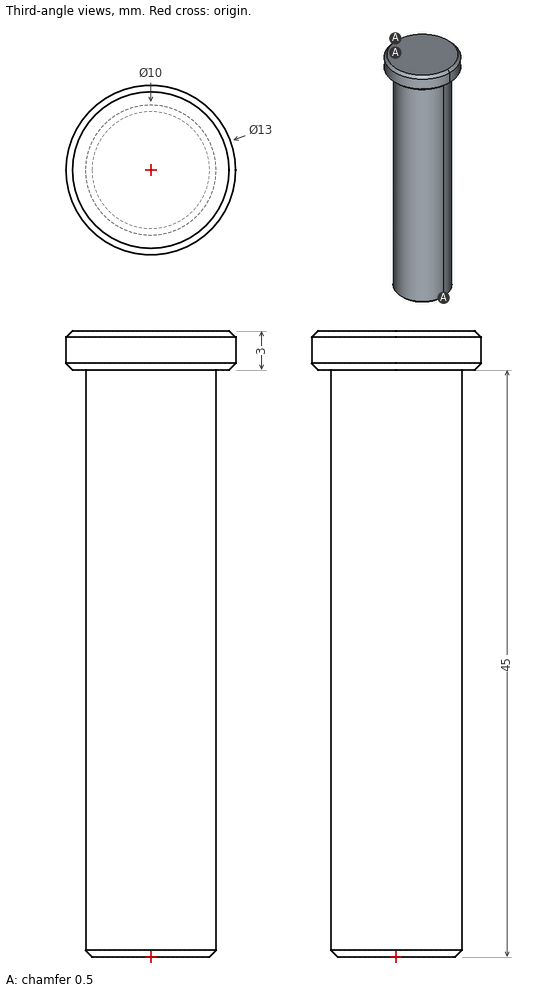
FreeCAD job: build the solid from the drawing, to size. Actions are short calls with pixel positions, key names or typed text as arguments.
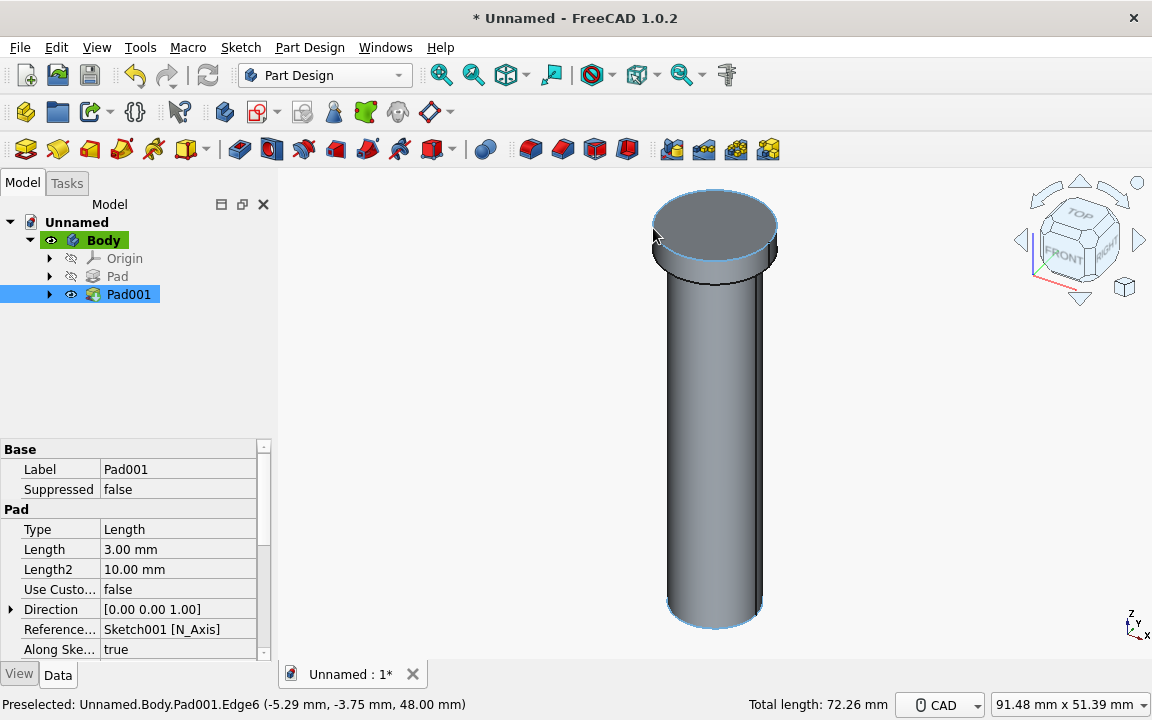
key(0)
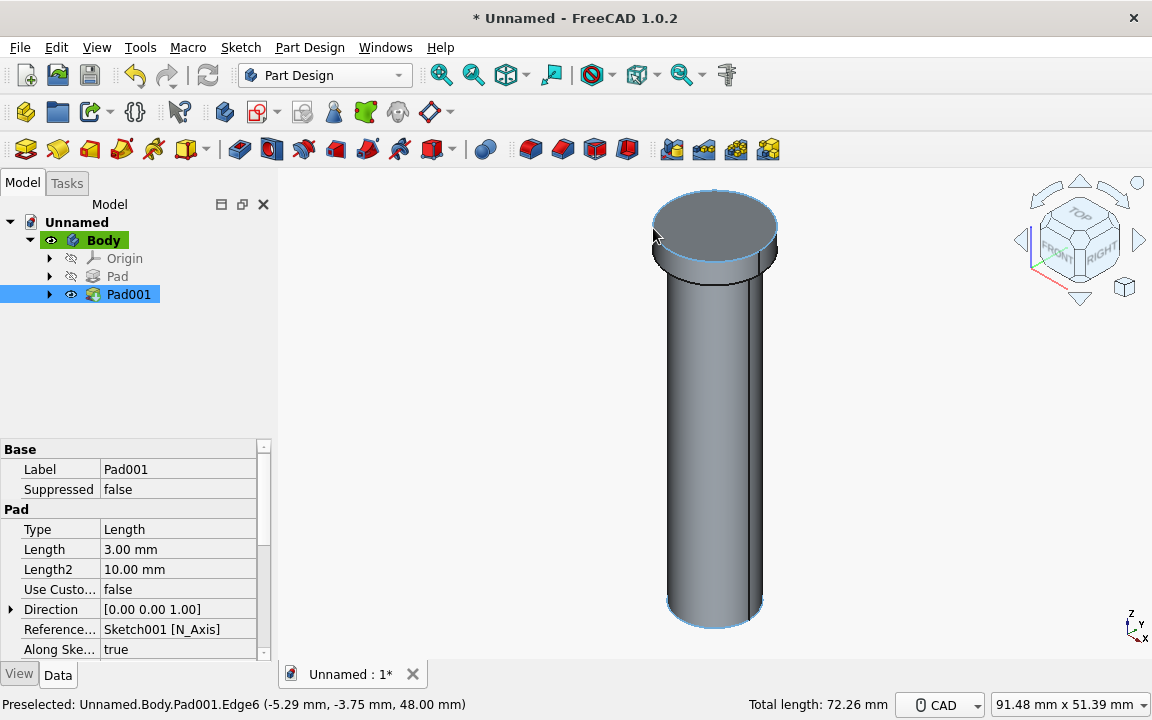
click(687, 281, ctrl)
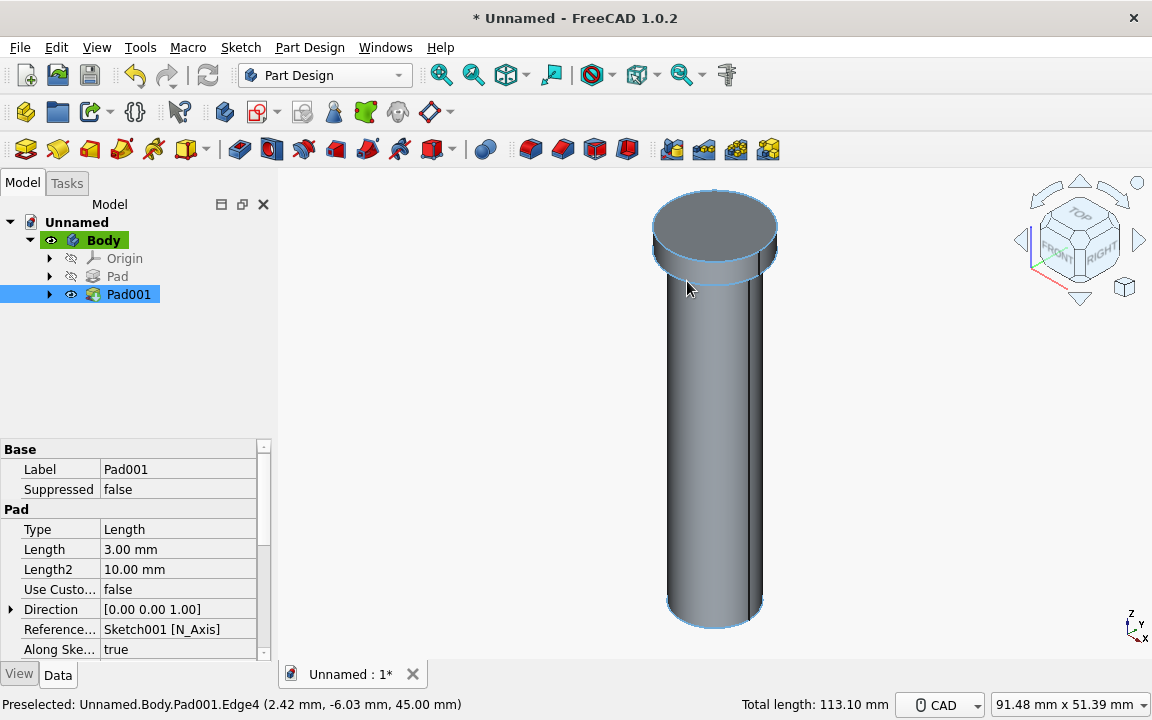
click(564, 150)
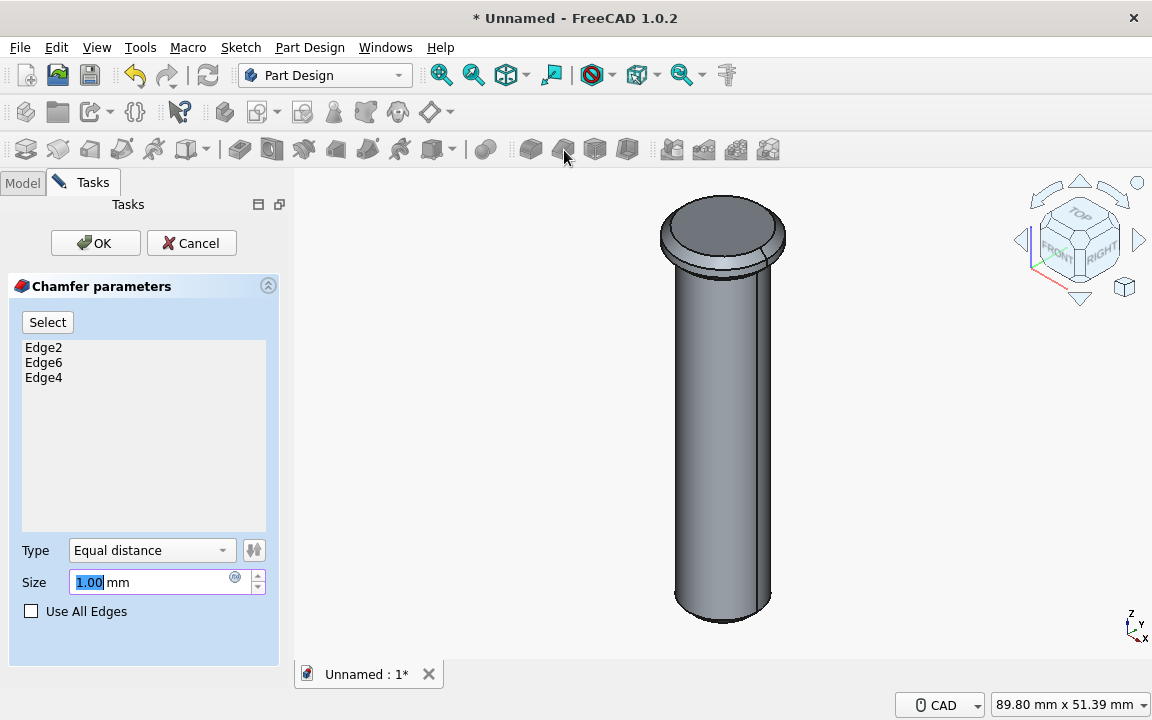
text(0.5)
key(Tab)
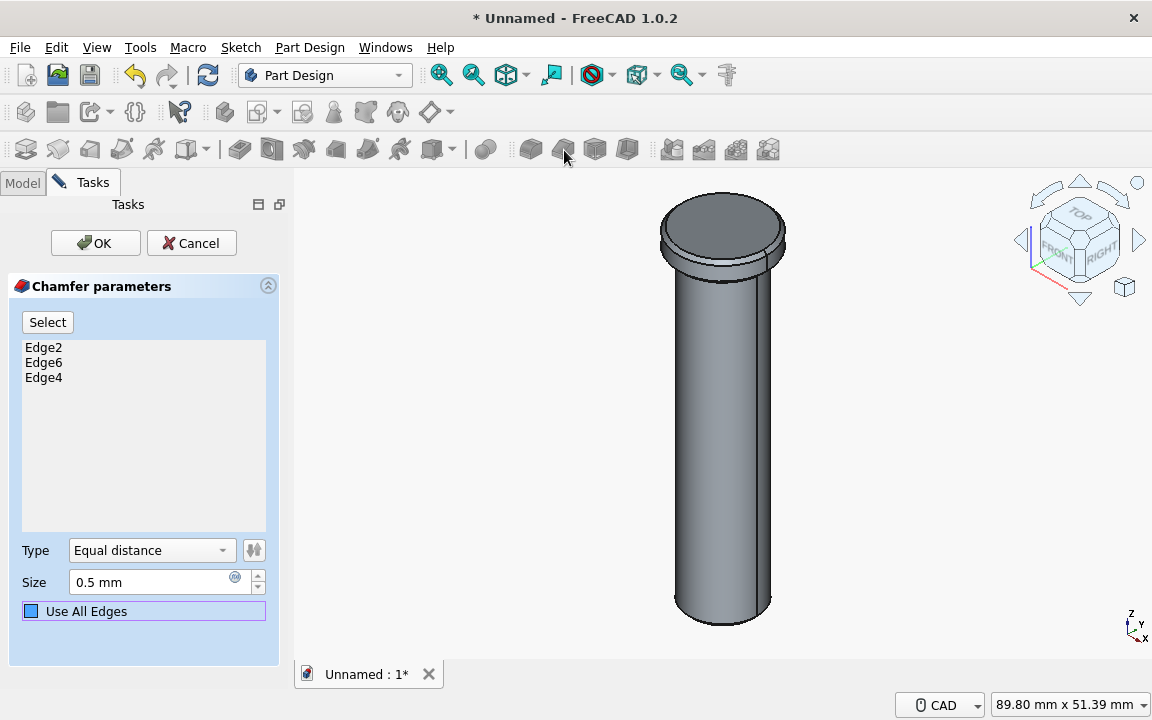
click(96, 243)